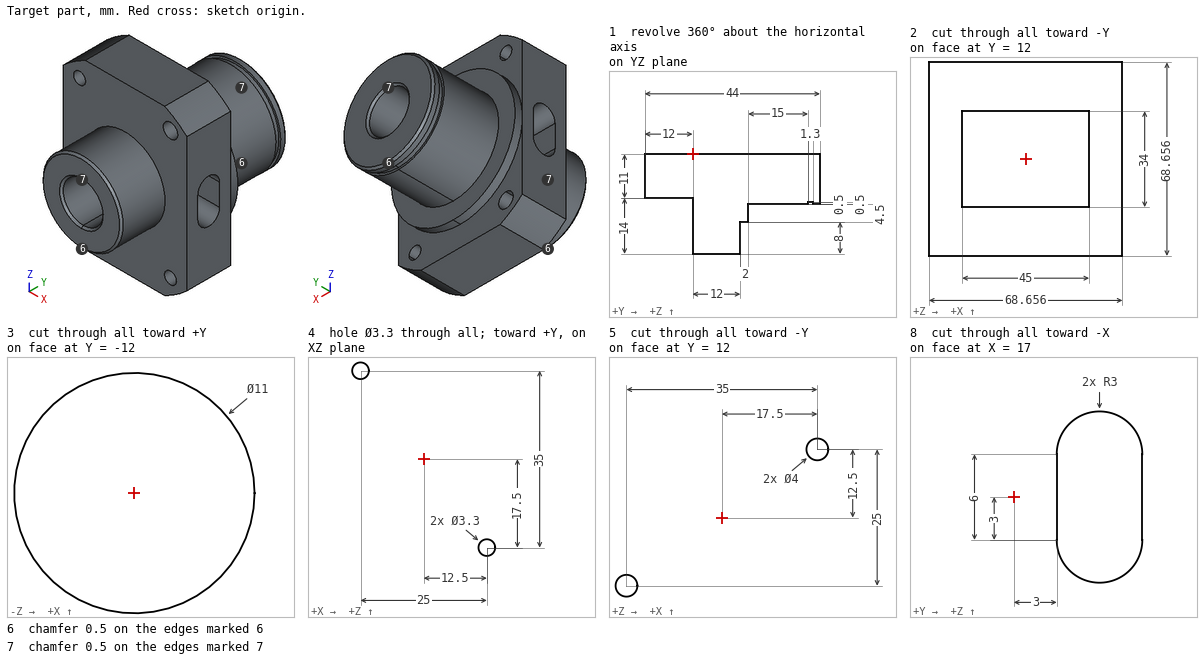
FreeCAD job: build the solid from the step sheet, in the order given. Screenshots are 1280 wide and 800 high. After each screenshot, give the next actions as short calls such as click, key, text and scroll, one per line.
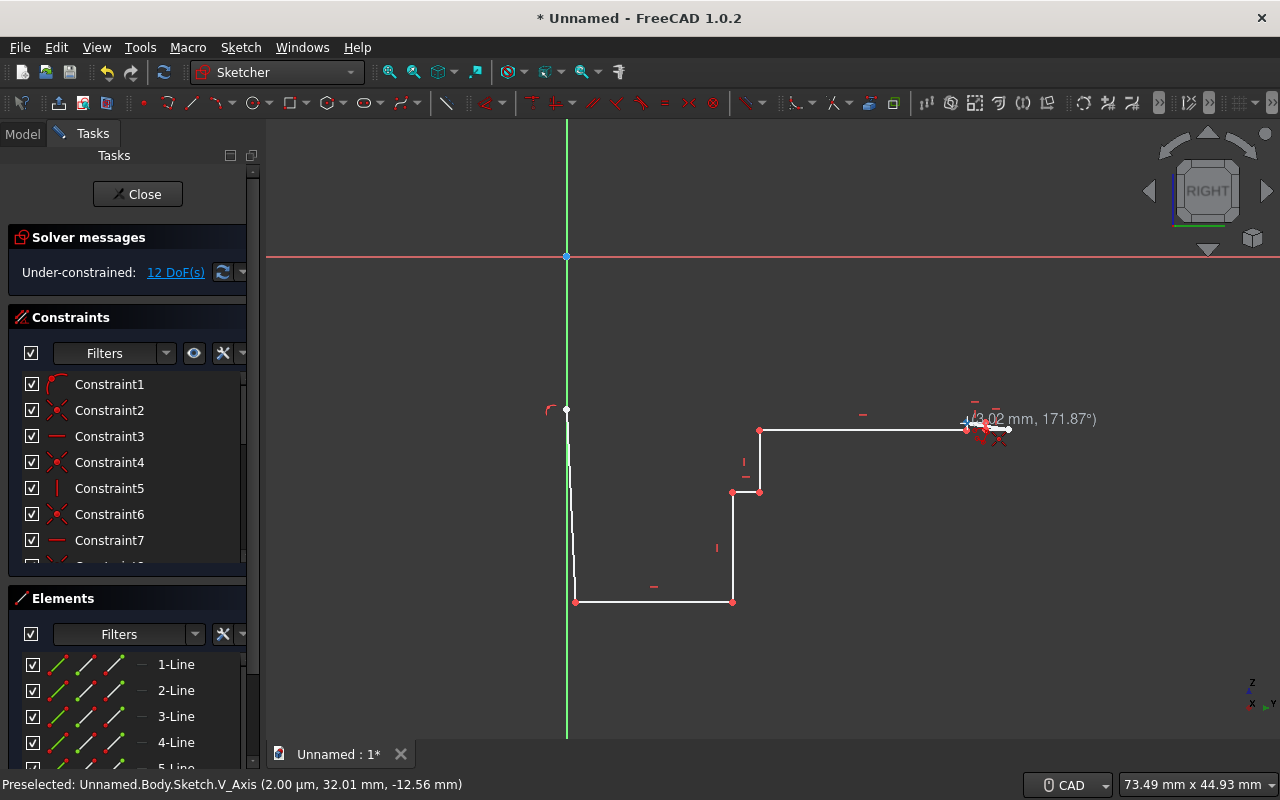
click(1009, 257)
click(401, 266)
click(401, 408)
click(567, 409)
key(Escape)
key(Escape)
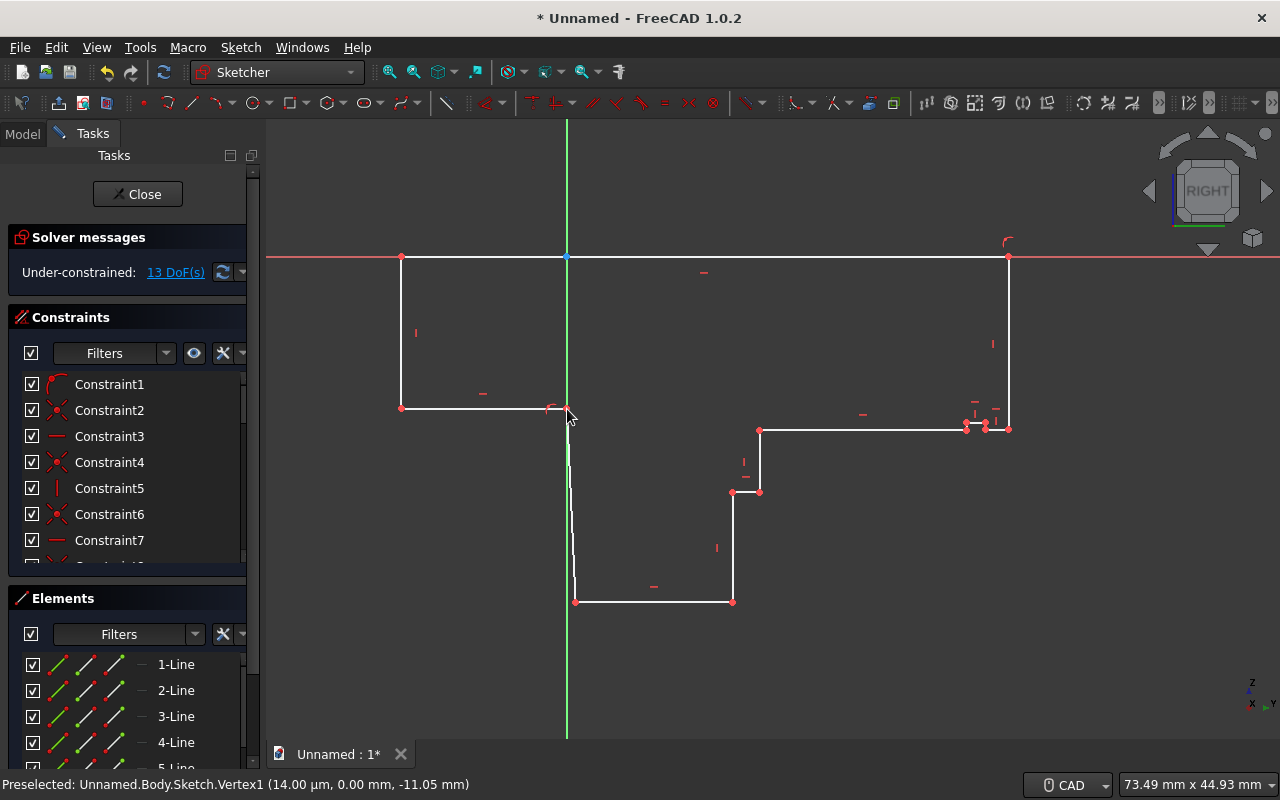
click(570, 467)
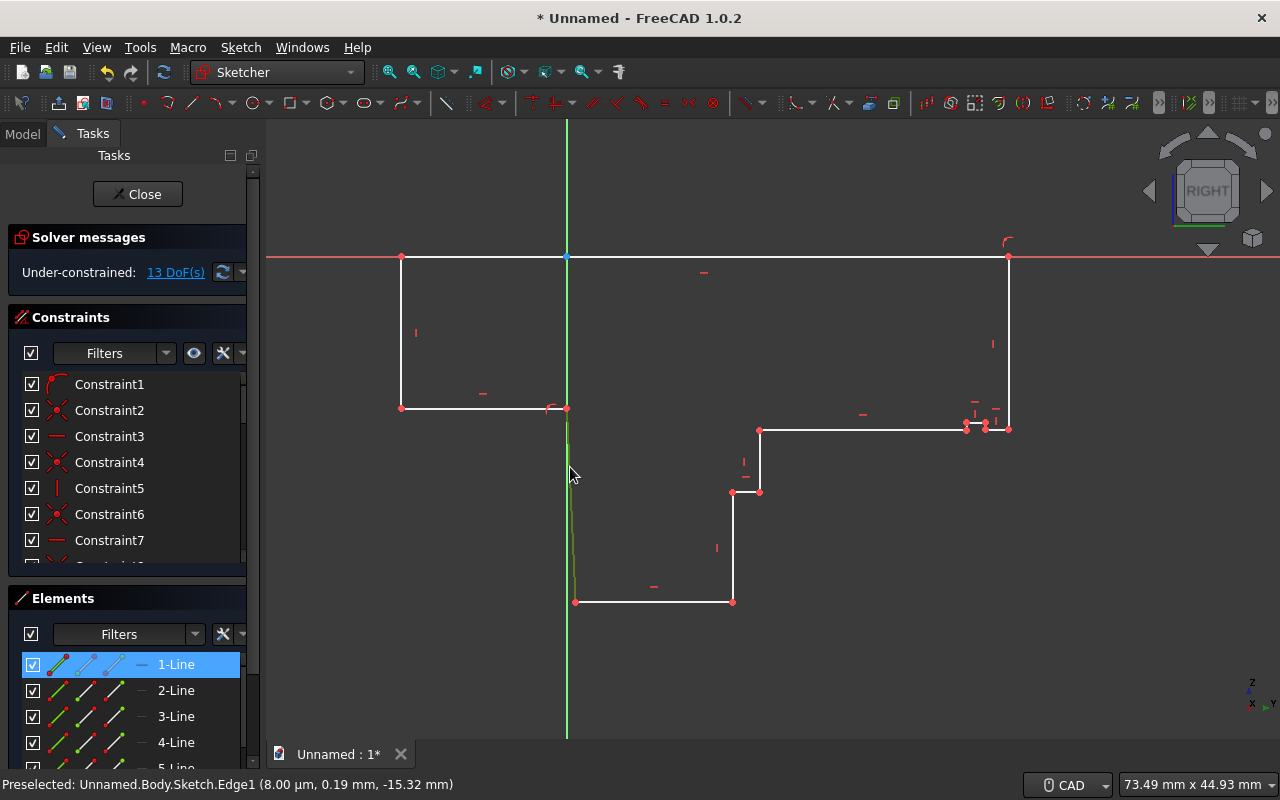
key(v)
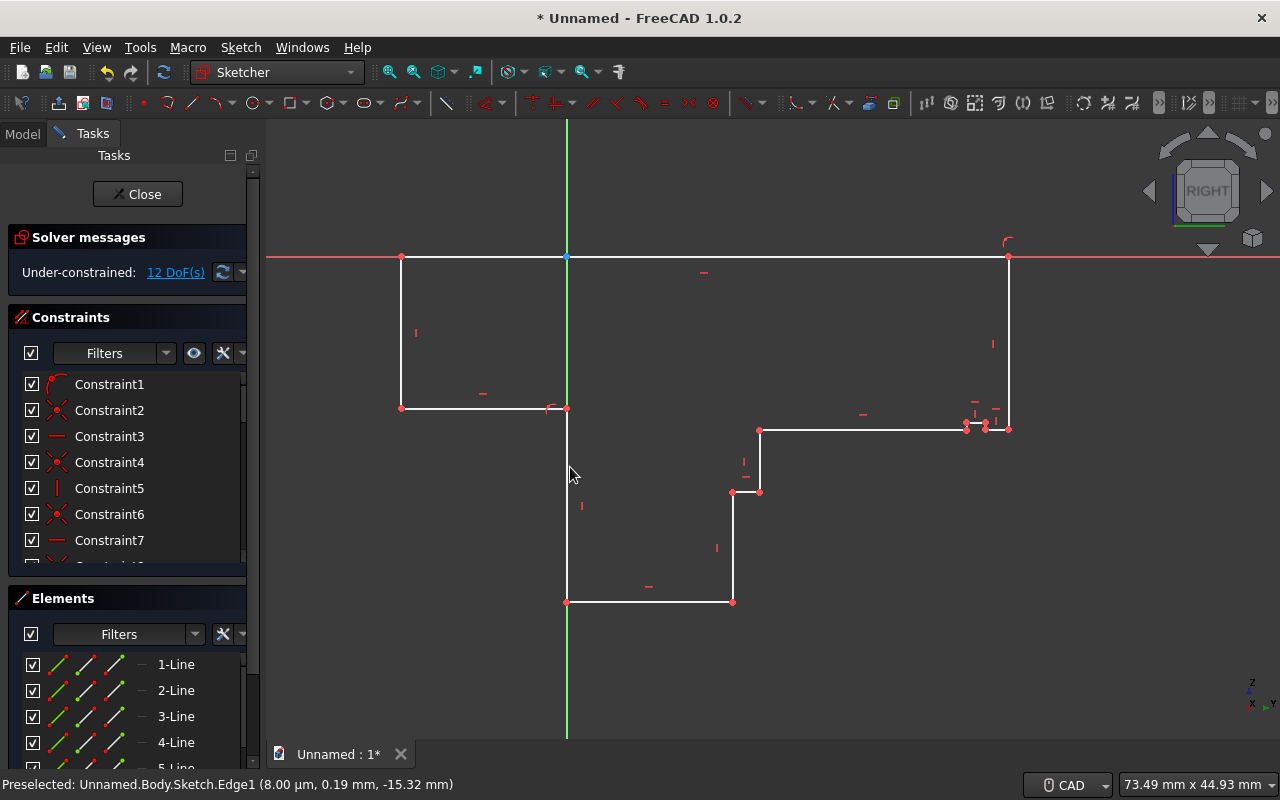
click(486, 104)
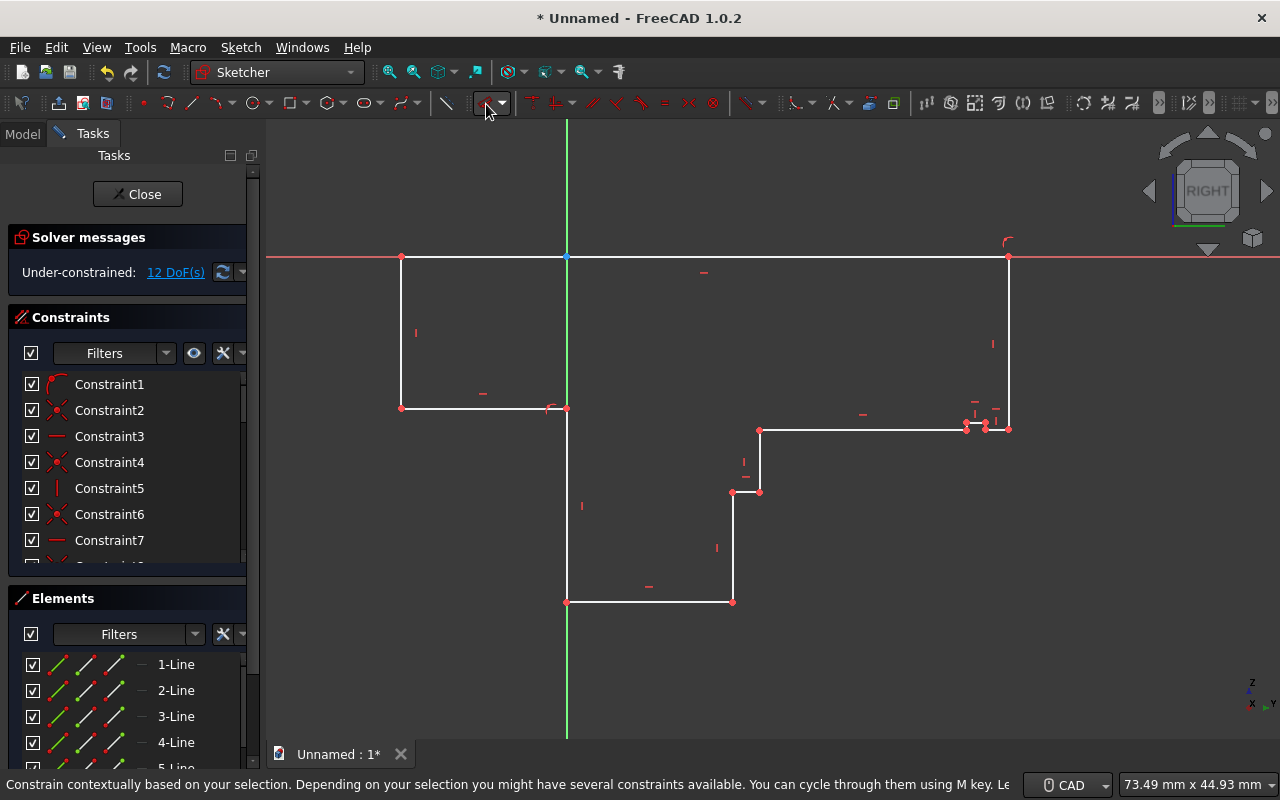
click(733, 569)
click(767, 547)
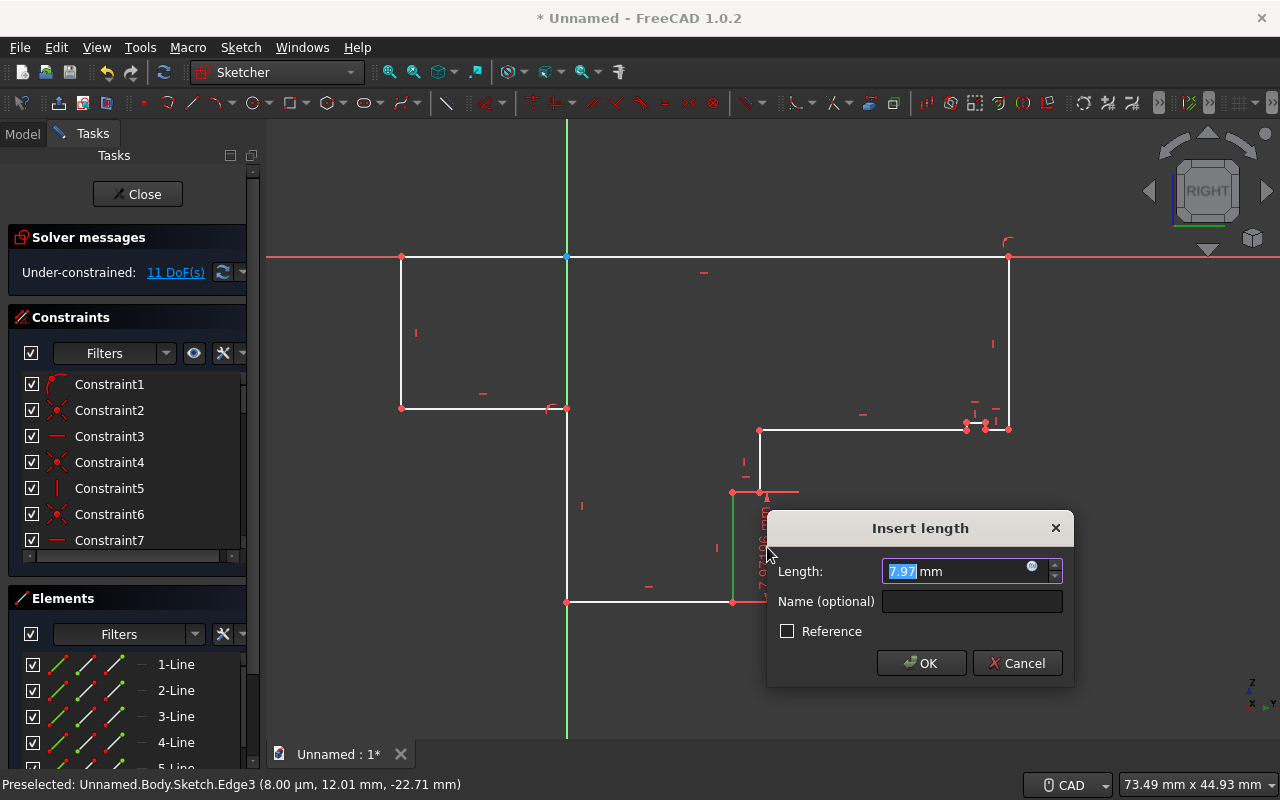
text(8)
key(Return)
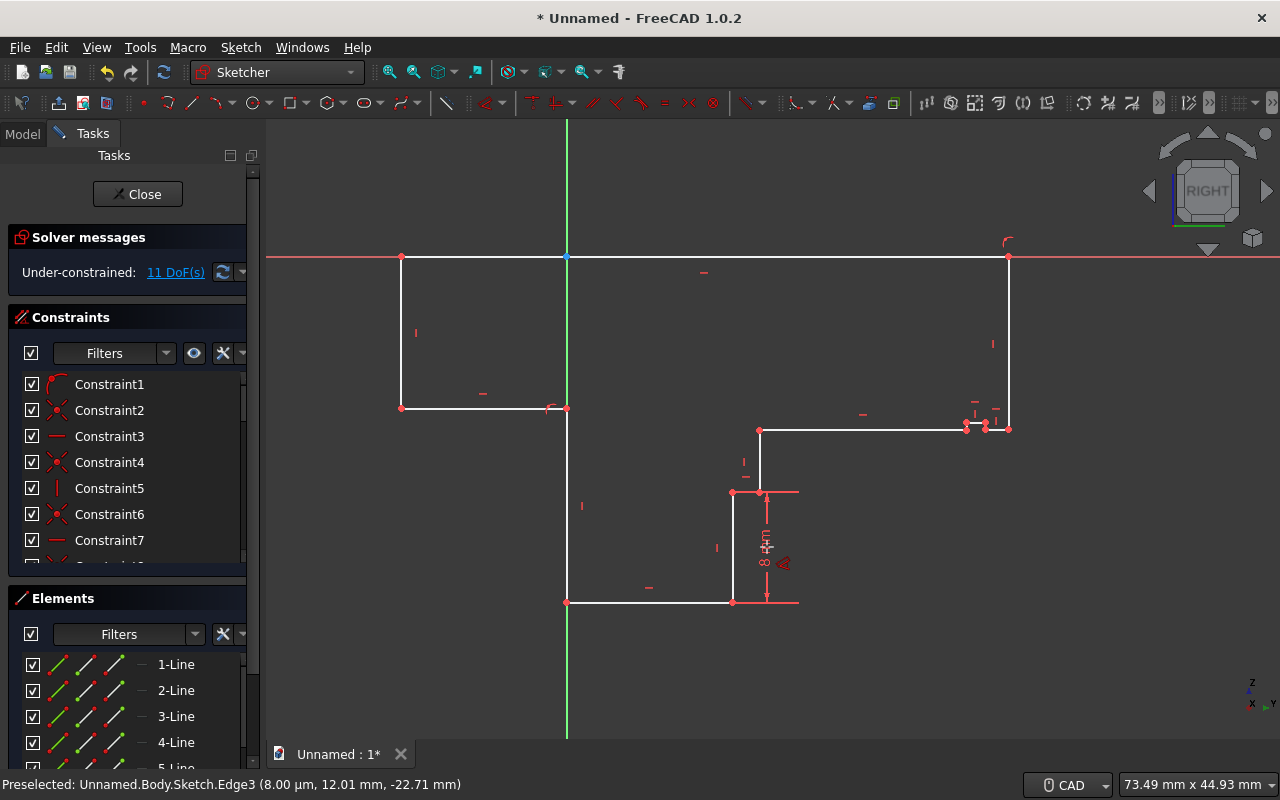
scroll(743, 492, up, 2)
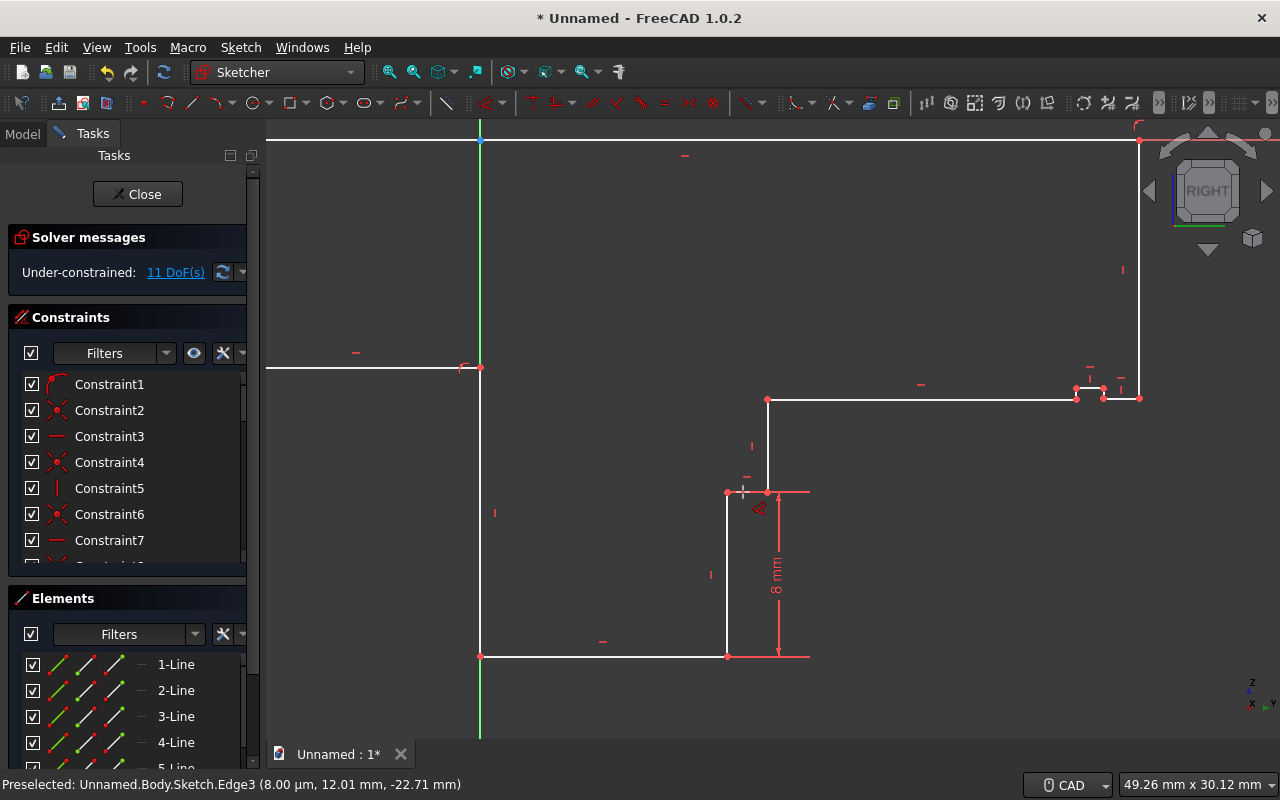
click(743, 492)
click(747, 526)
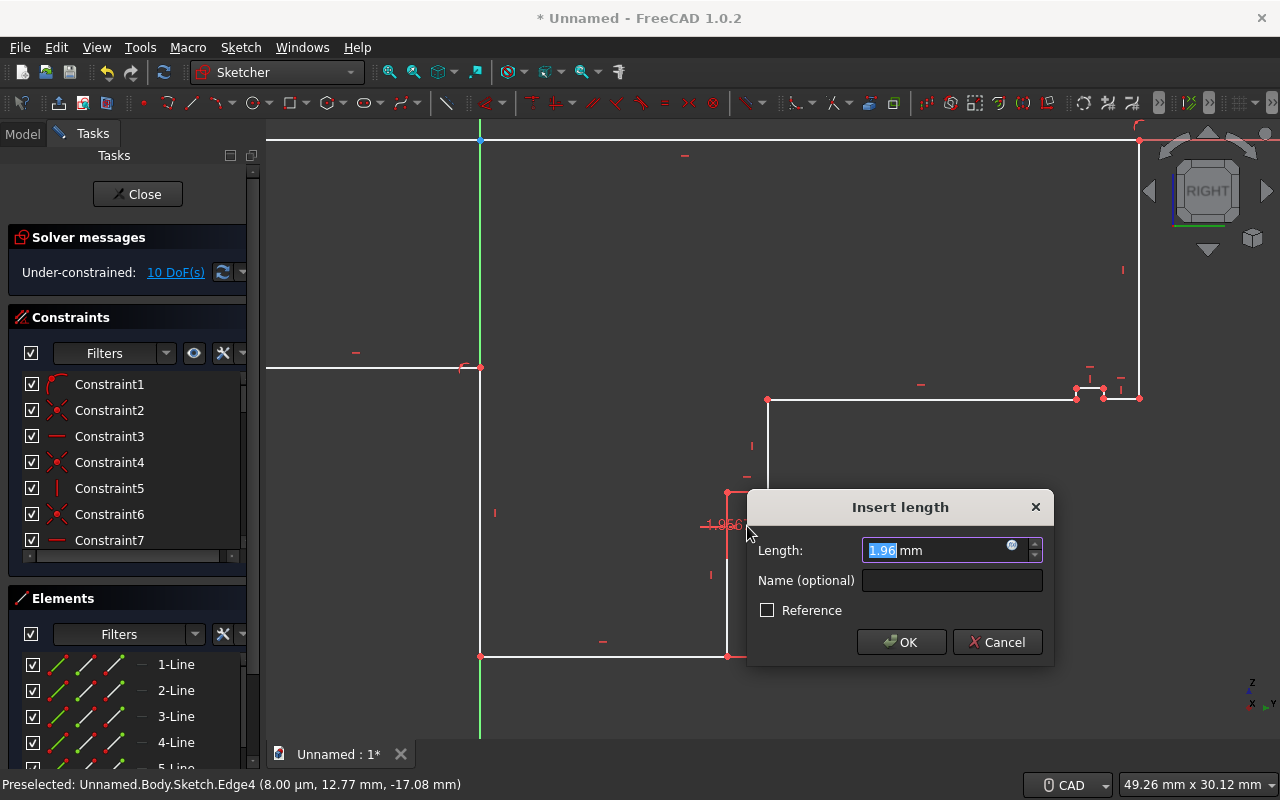
text(2)
key(Return)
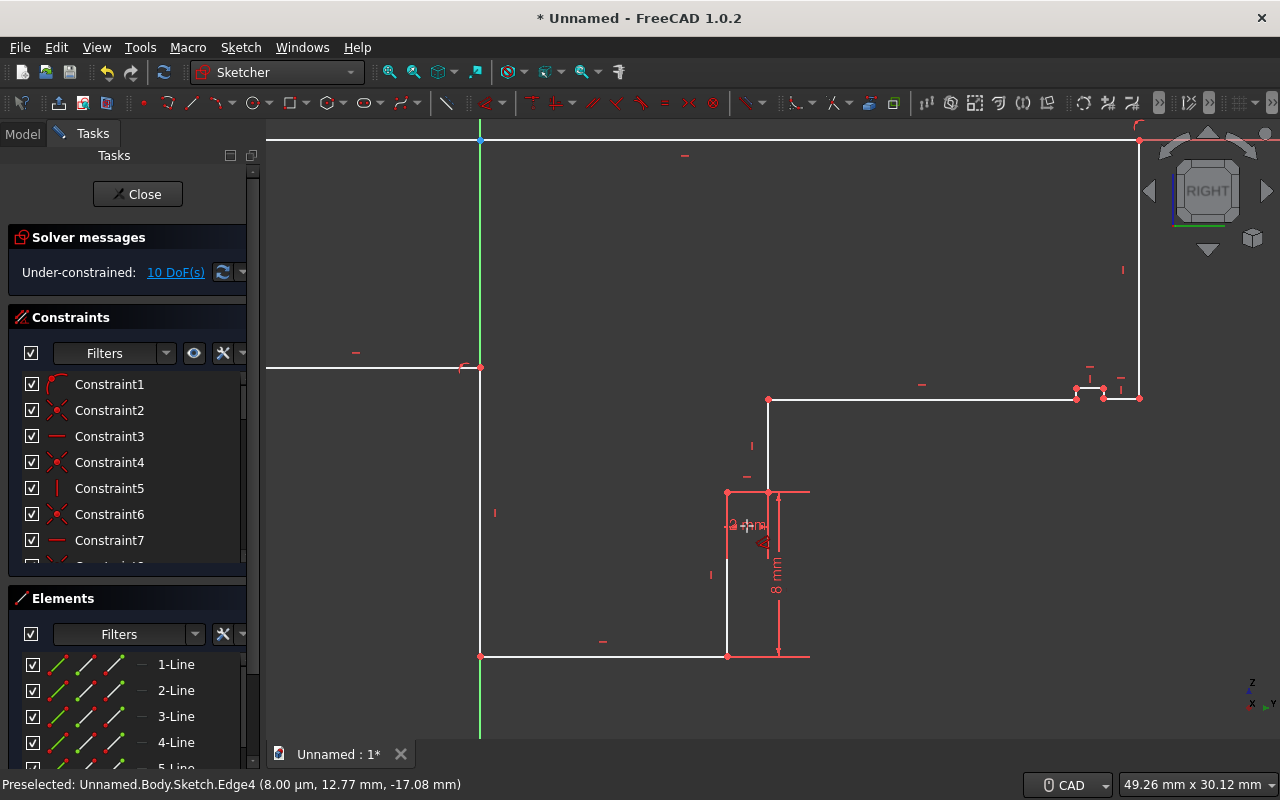
click(480, 455)
click(446, 512)